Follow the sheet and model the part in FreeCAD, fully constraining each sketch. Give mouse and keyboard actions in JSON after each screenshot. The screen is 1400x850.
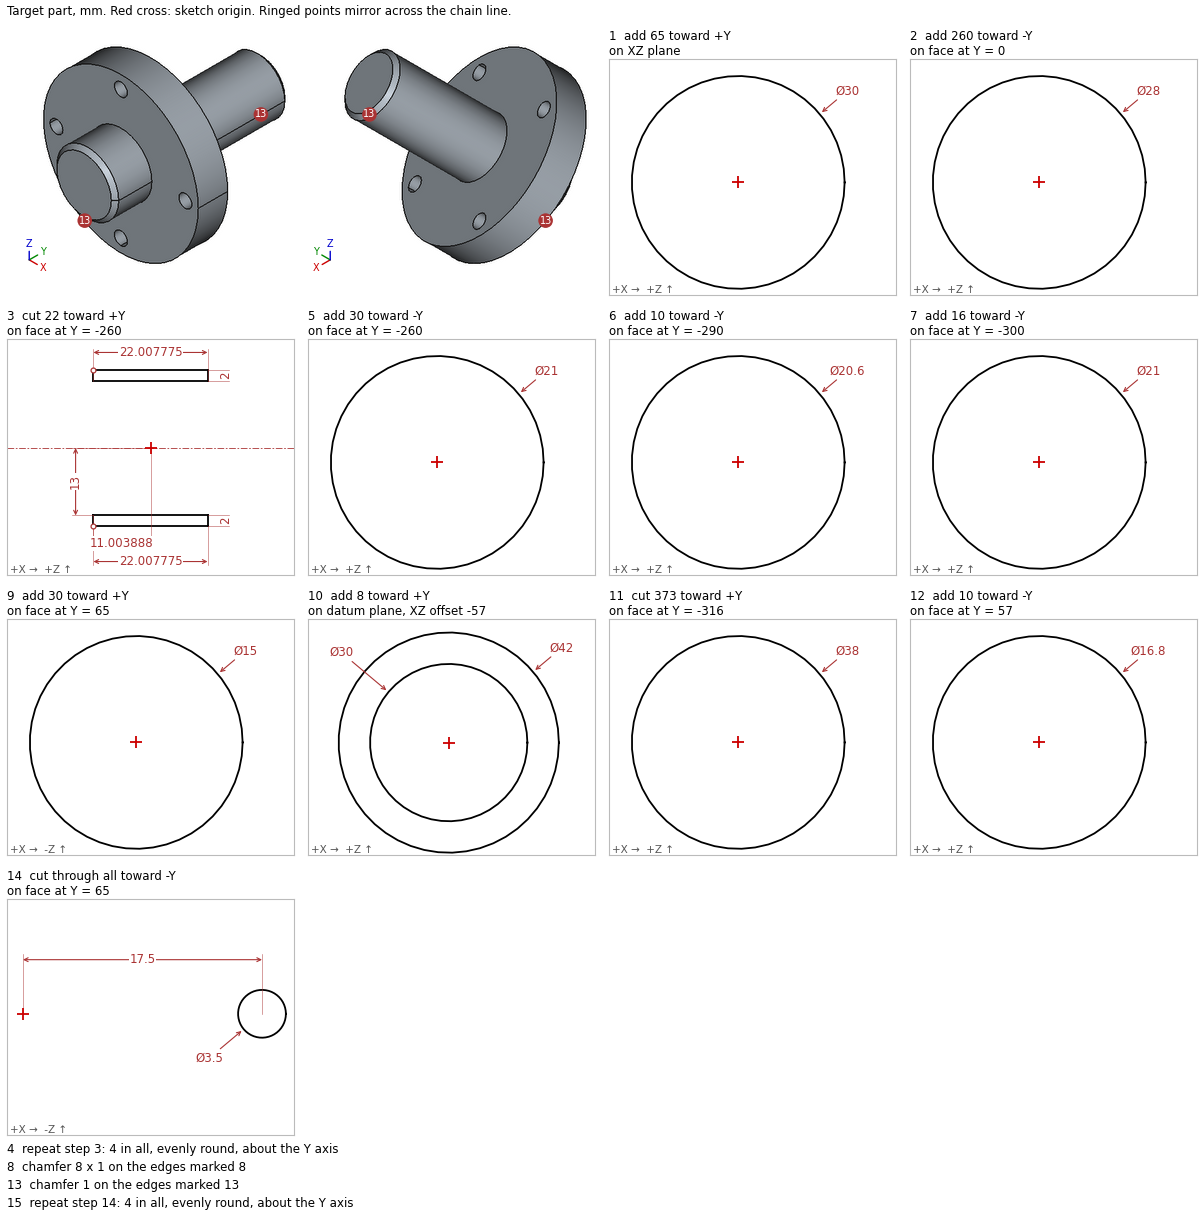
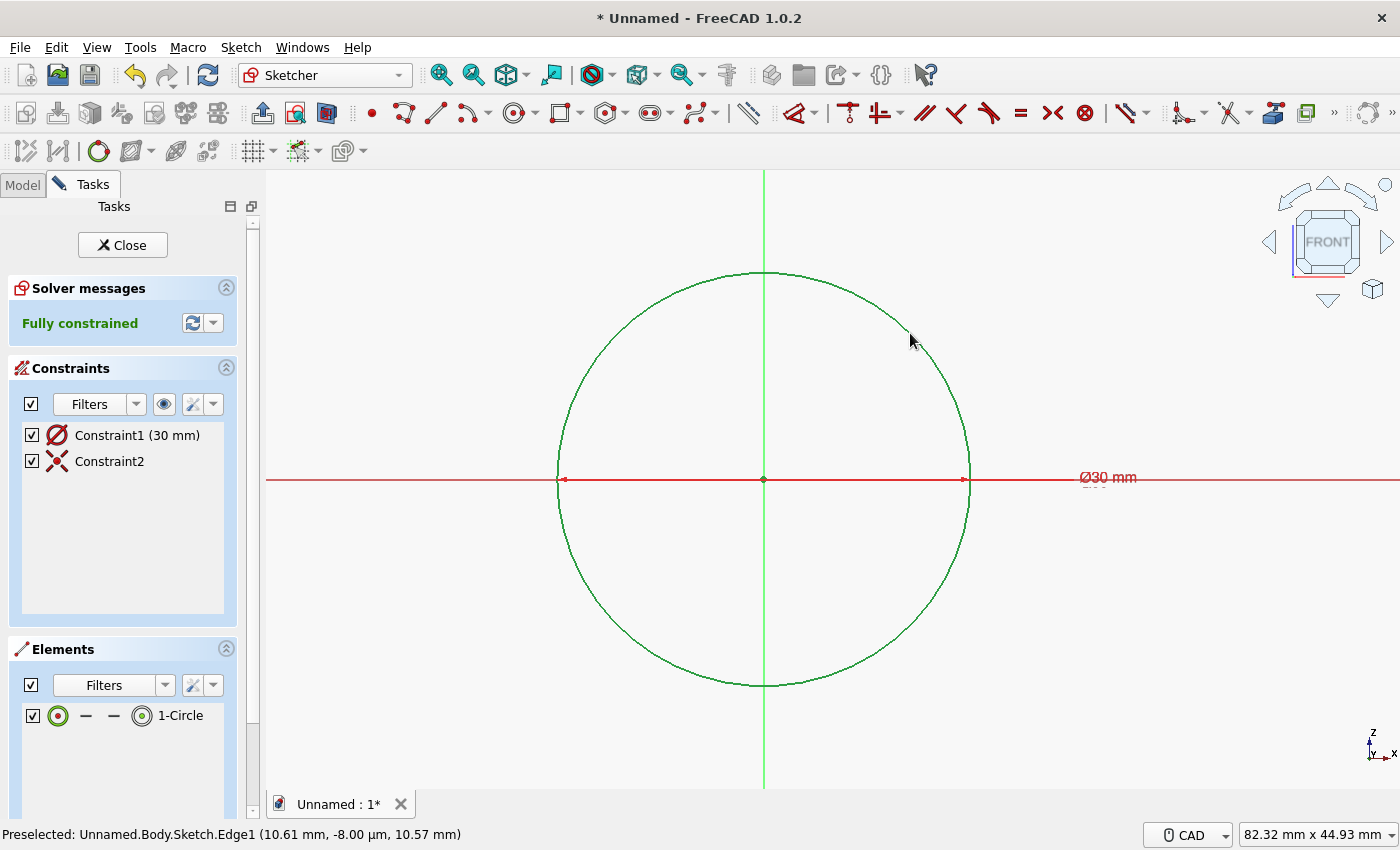
{"action": "left_click", "coordinate": [123, 245]}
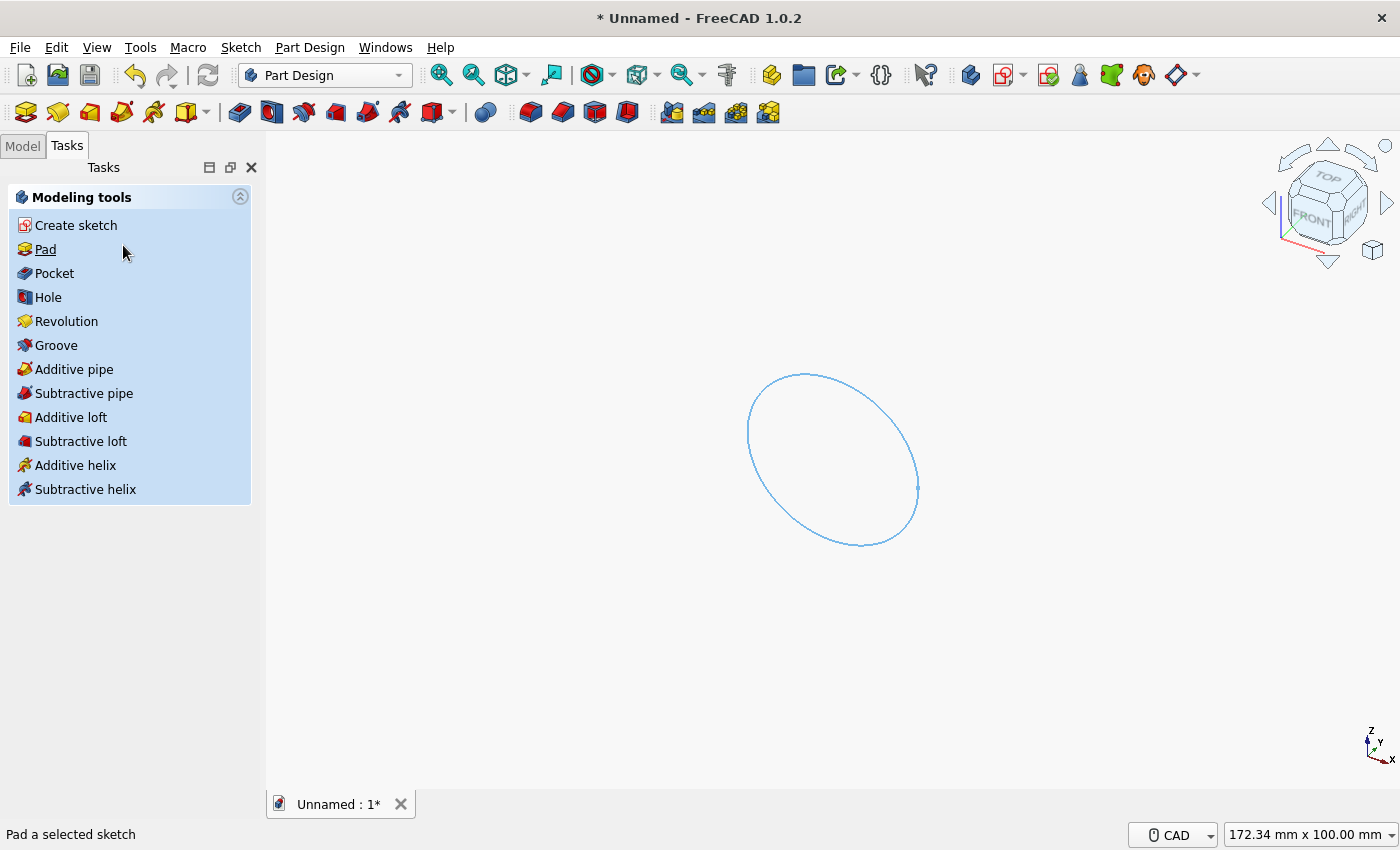
{"action": "left_click", "coordinate": [26, 112]}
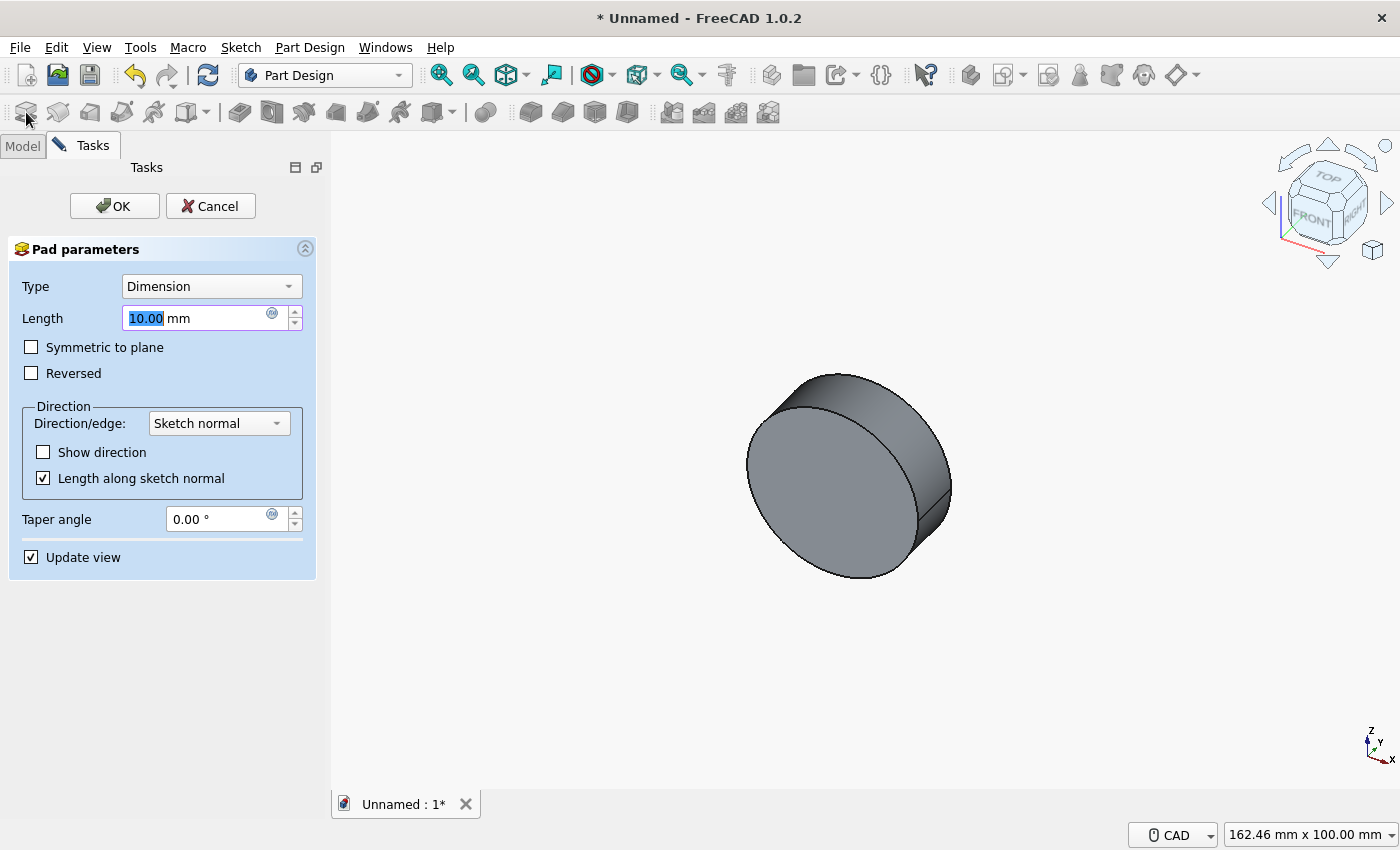
{"action": "type", "text": "65"}
{"action": "key", "text": "Tab"}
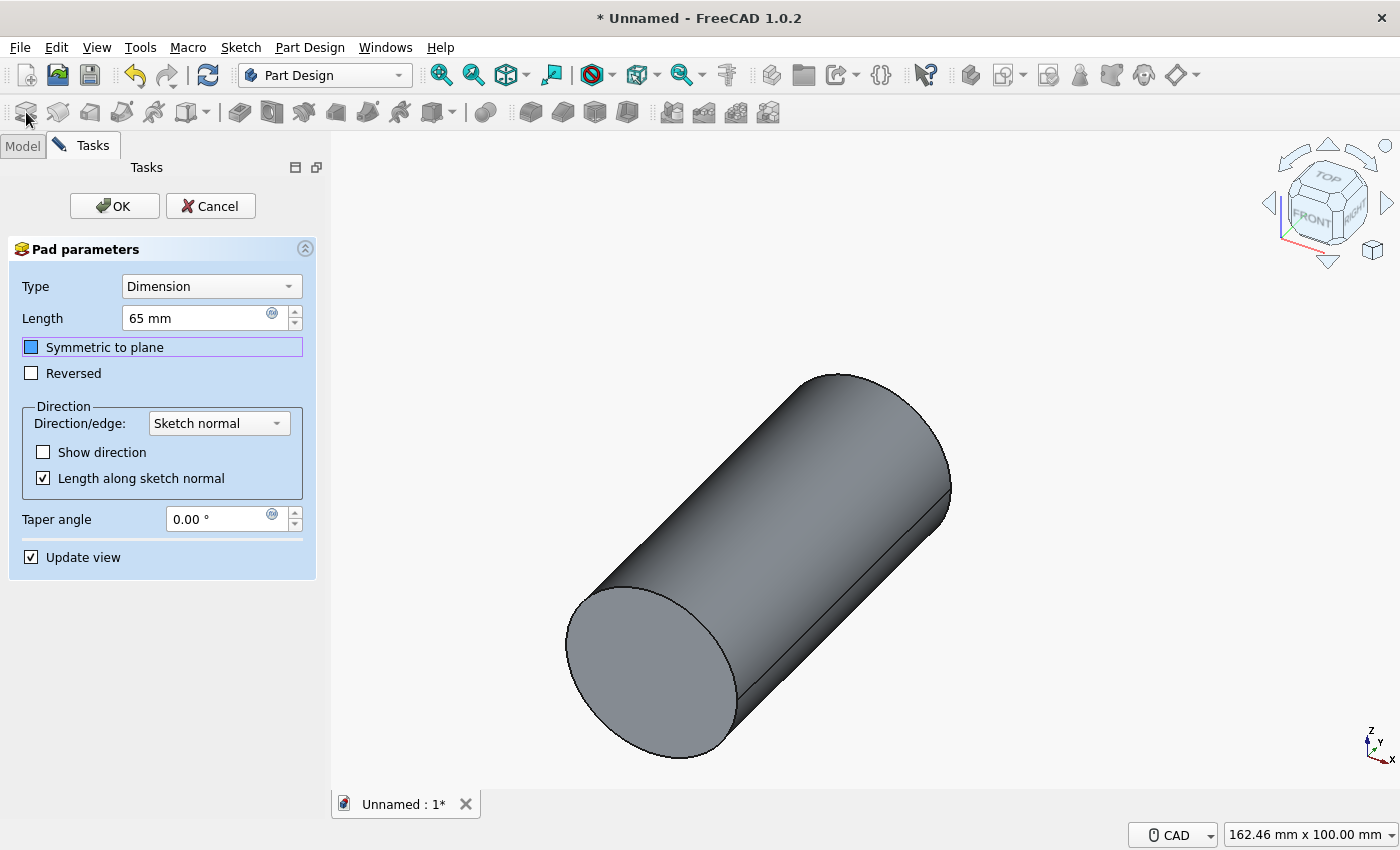
{"action": "left_click", "coordinate": [30, 373]}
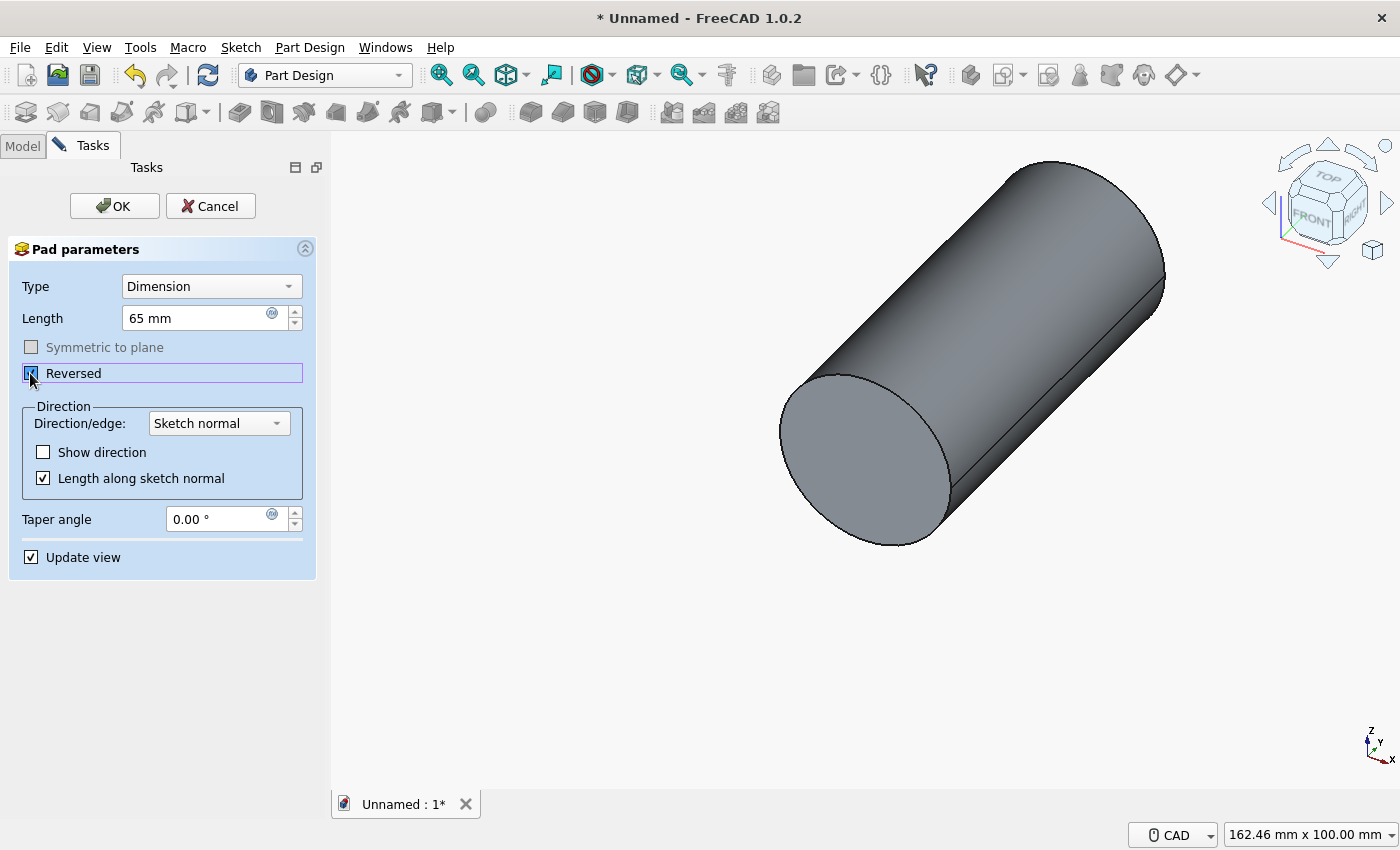
{"action": "left_click", "coordinate": [115, 206]}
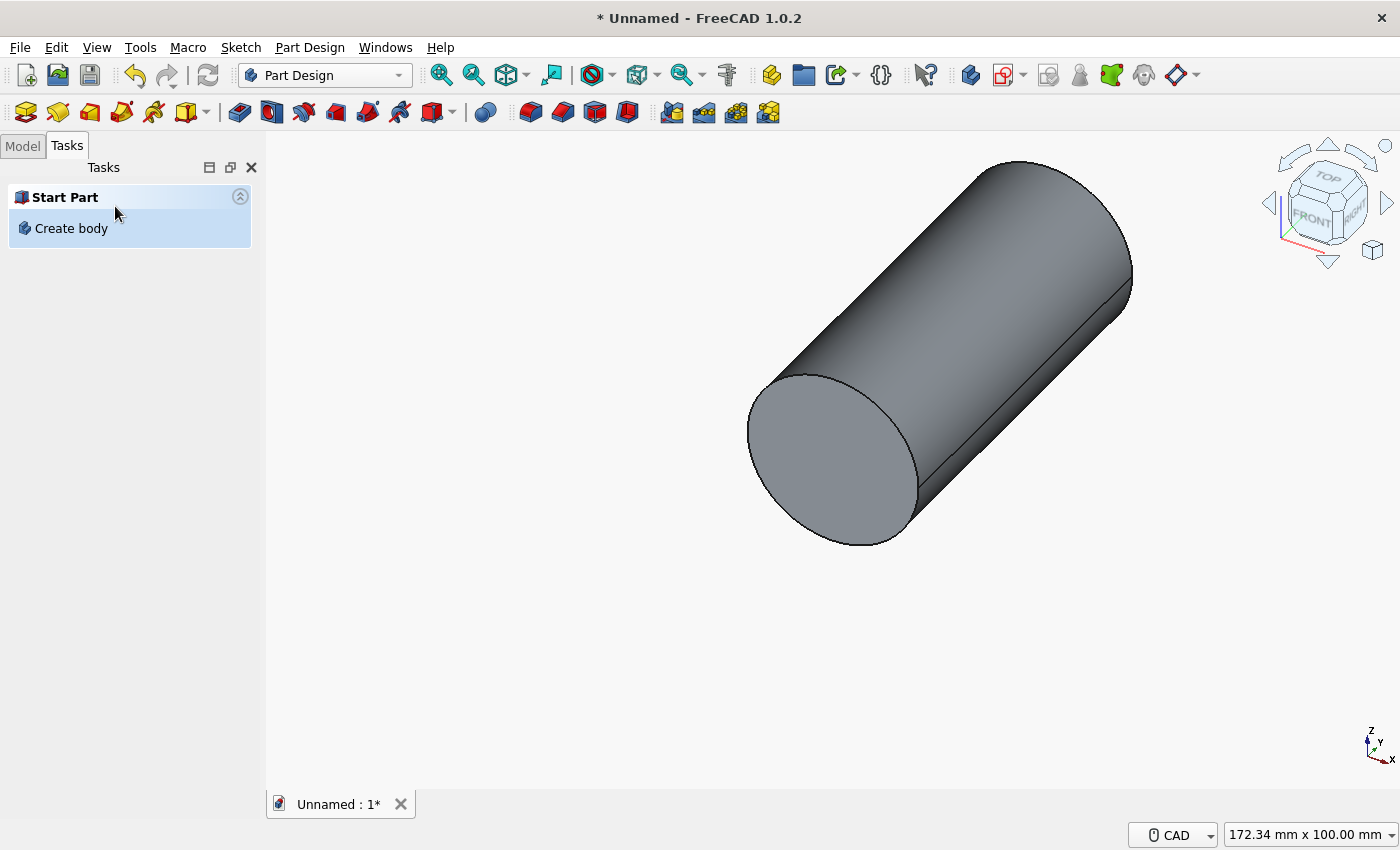
{"action": "left_click", "coordinate": [833, 459]}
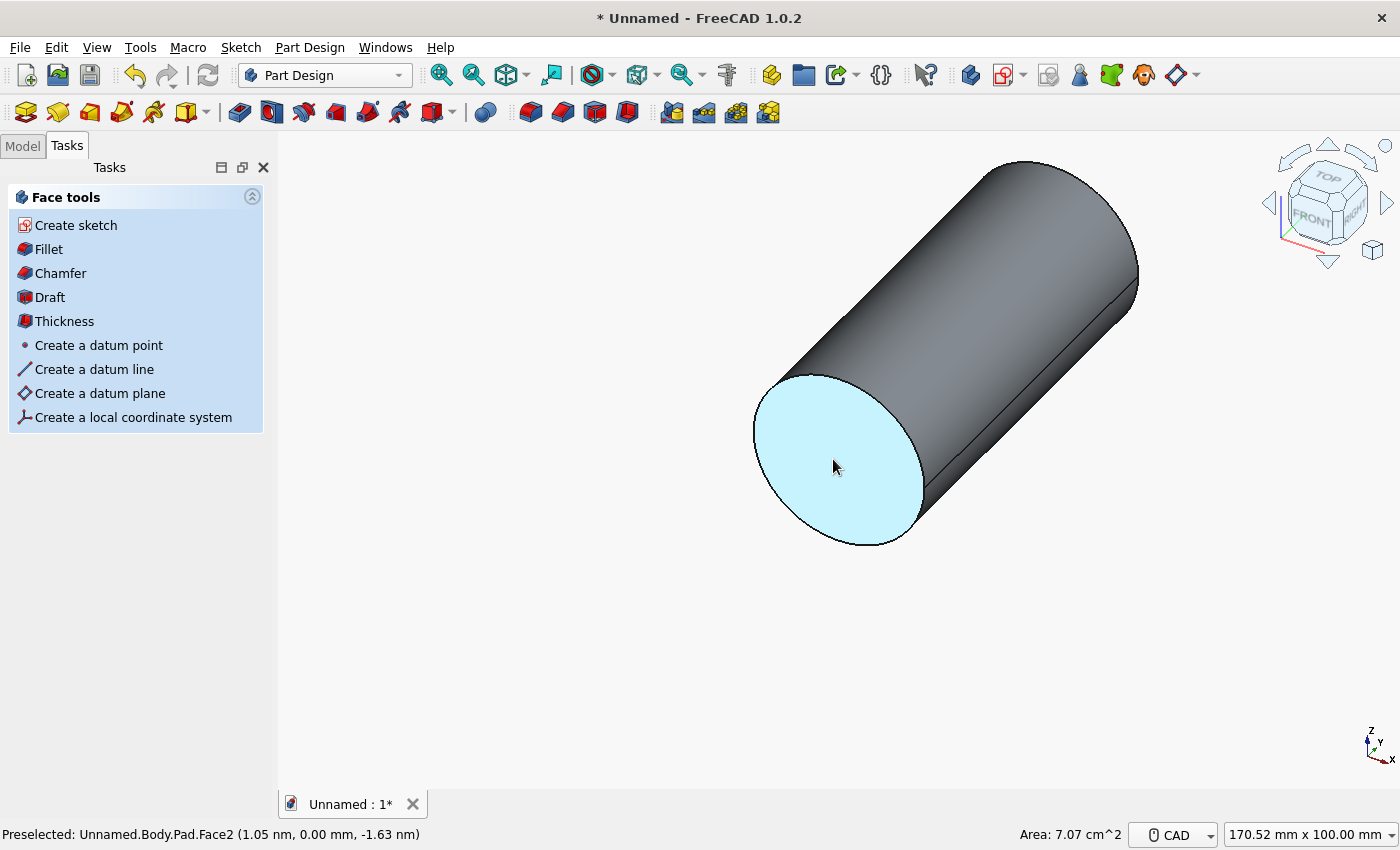
{"action": "left_click", "coordinate": [1004, 76]}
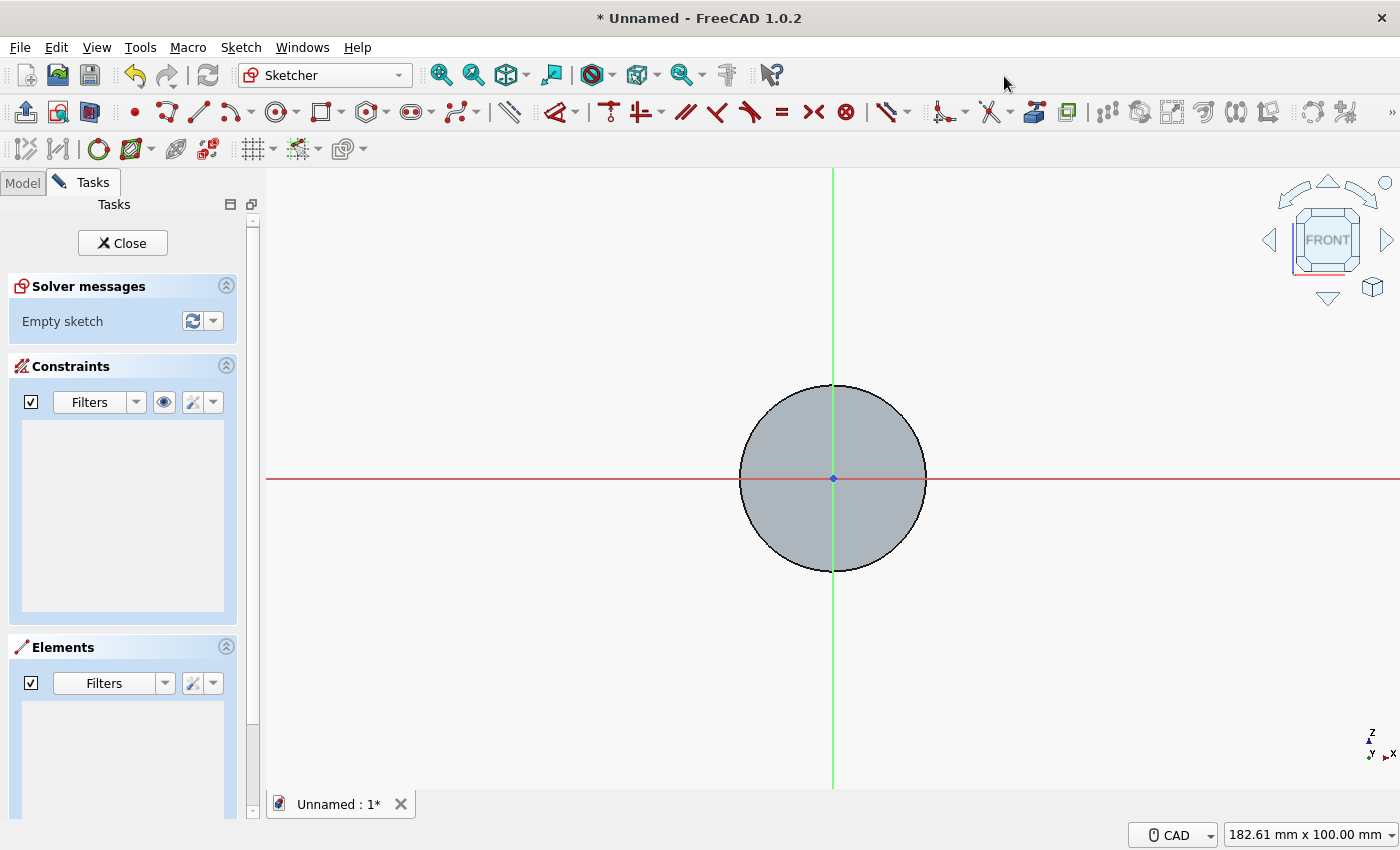
{"action": "scroll", "coordinate": [889, 478], "scroll_direction": "up", "scroll_amount": 4}